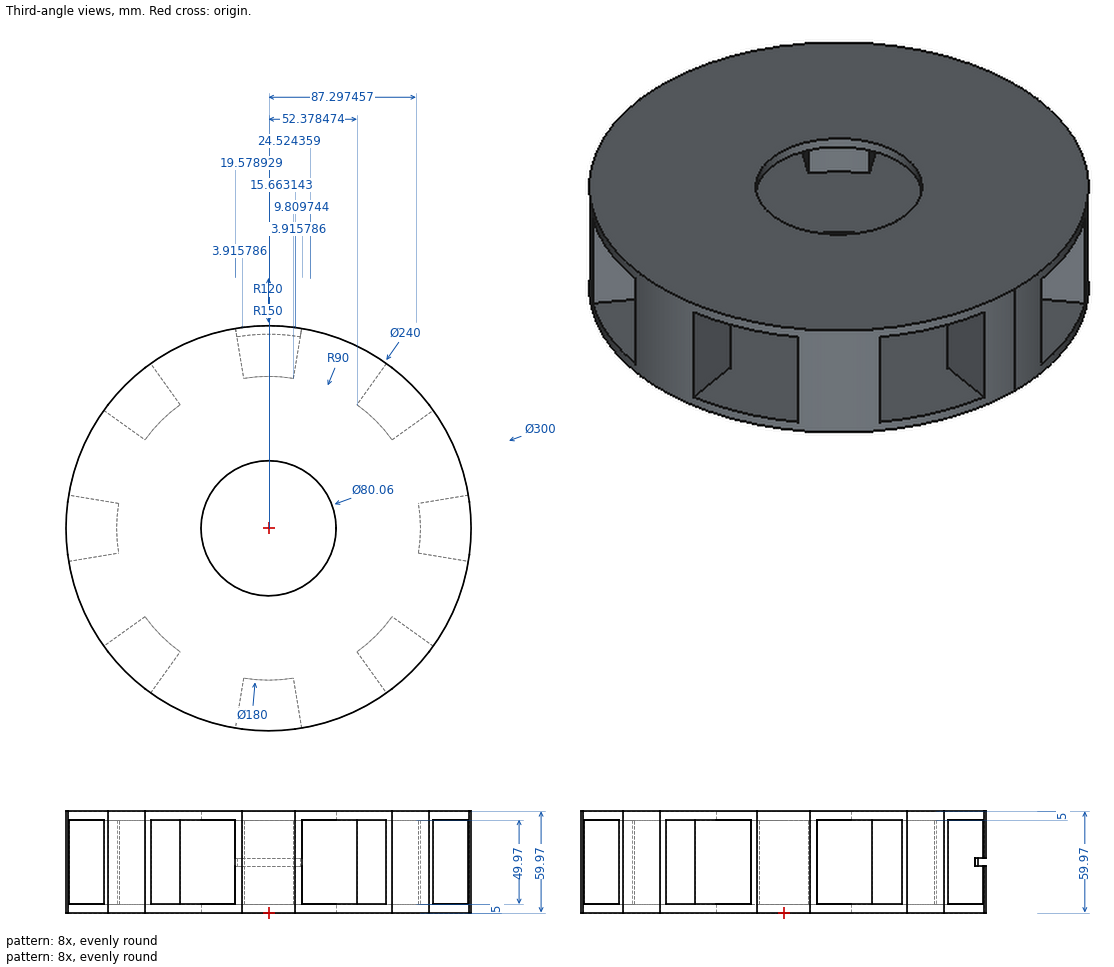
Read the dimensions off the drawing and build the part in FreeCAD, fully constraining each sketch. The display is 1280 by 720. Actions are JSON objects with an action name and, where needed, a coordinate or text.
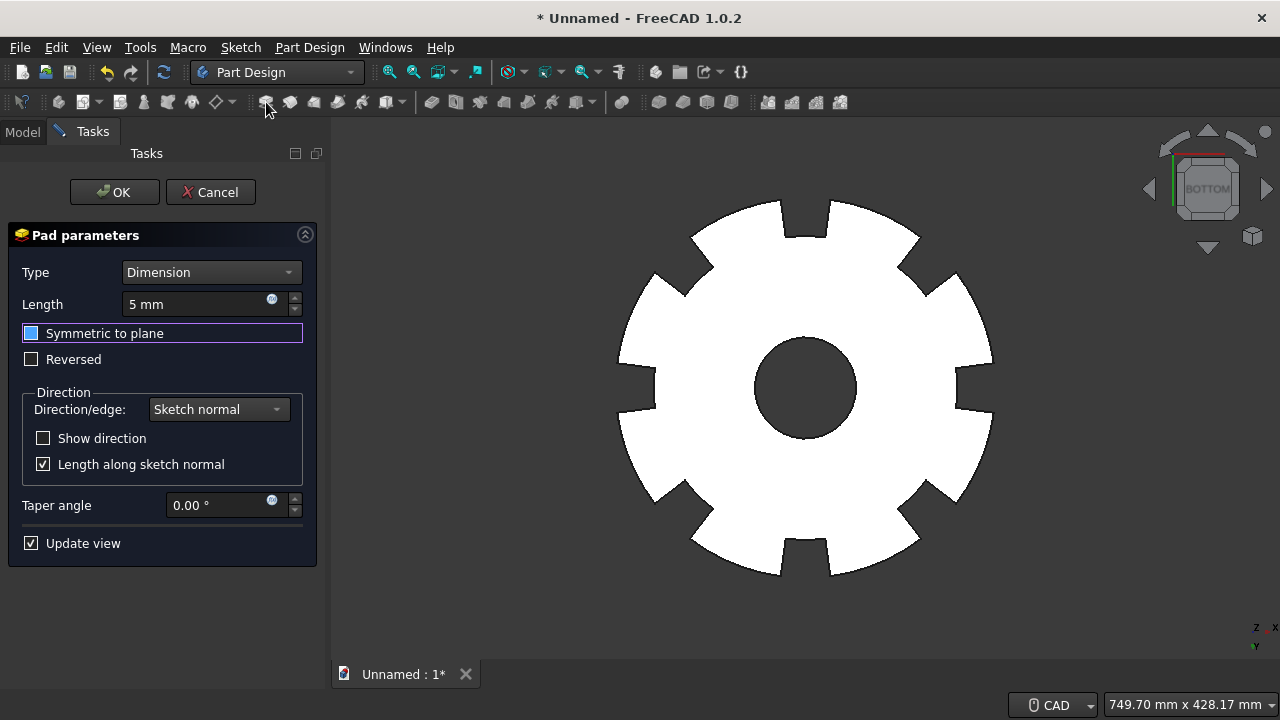
{"action": "left_click", "coordinate": [115, 192]}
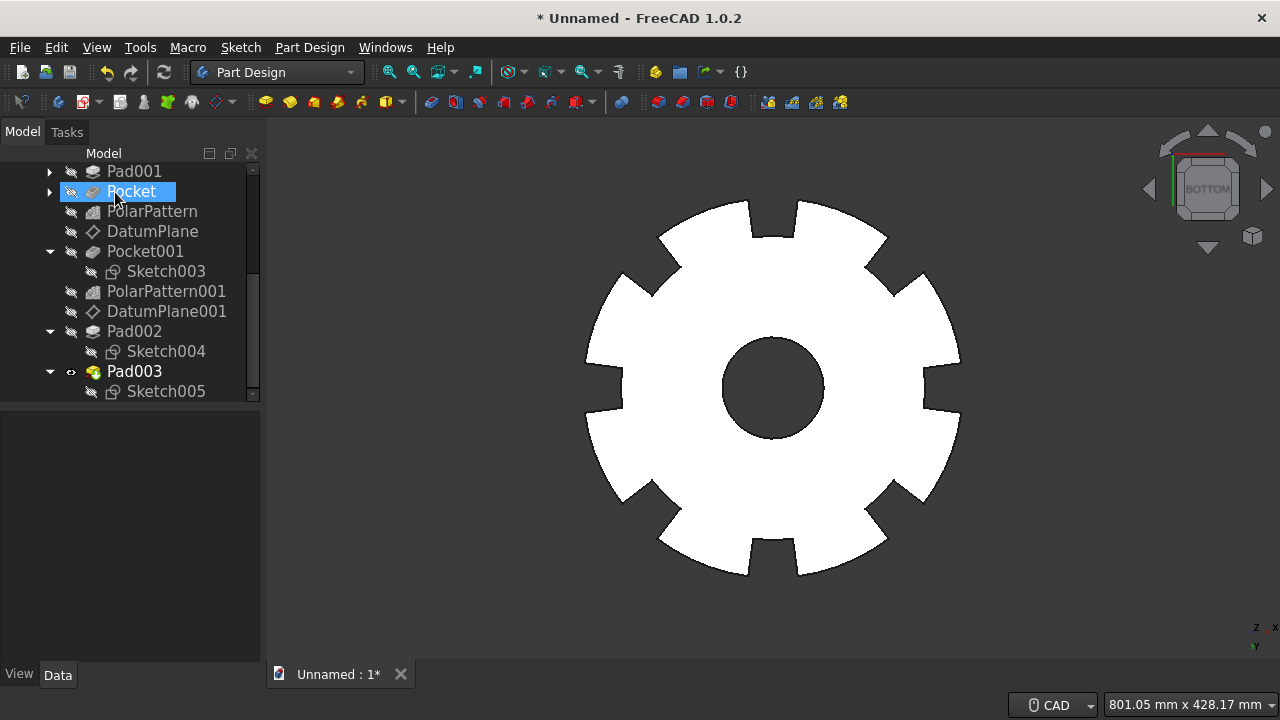
{"action": "left_click", "coordinate": [773, 495]}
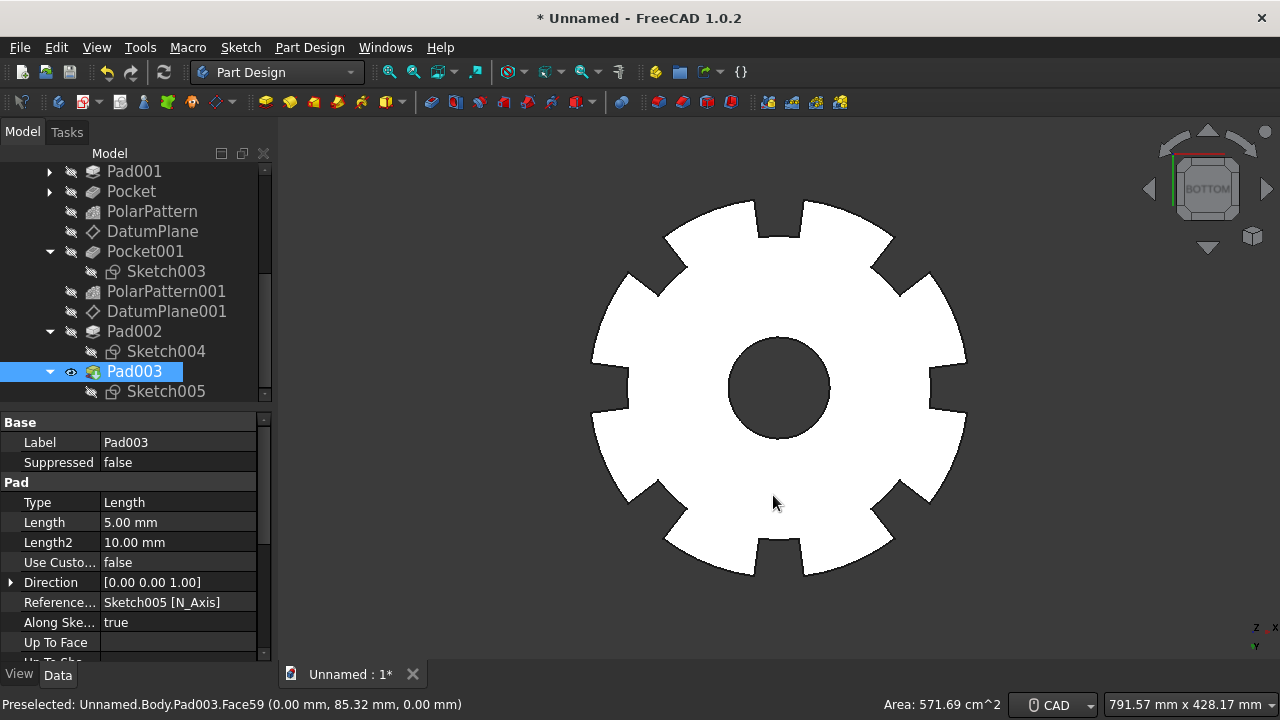
{"action": "left_click", "coordinate": [84, 102]}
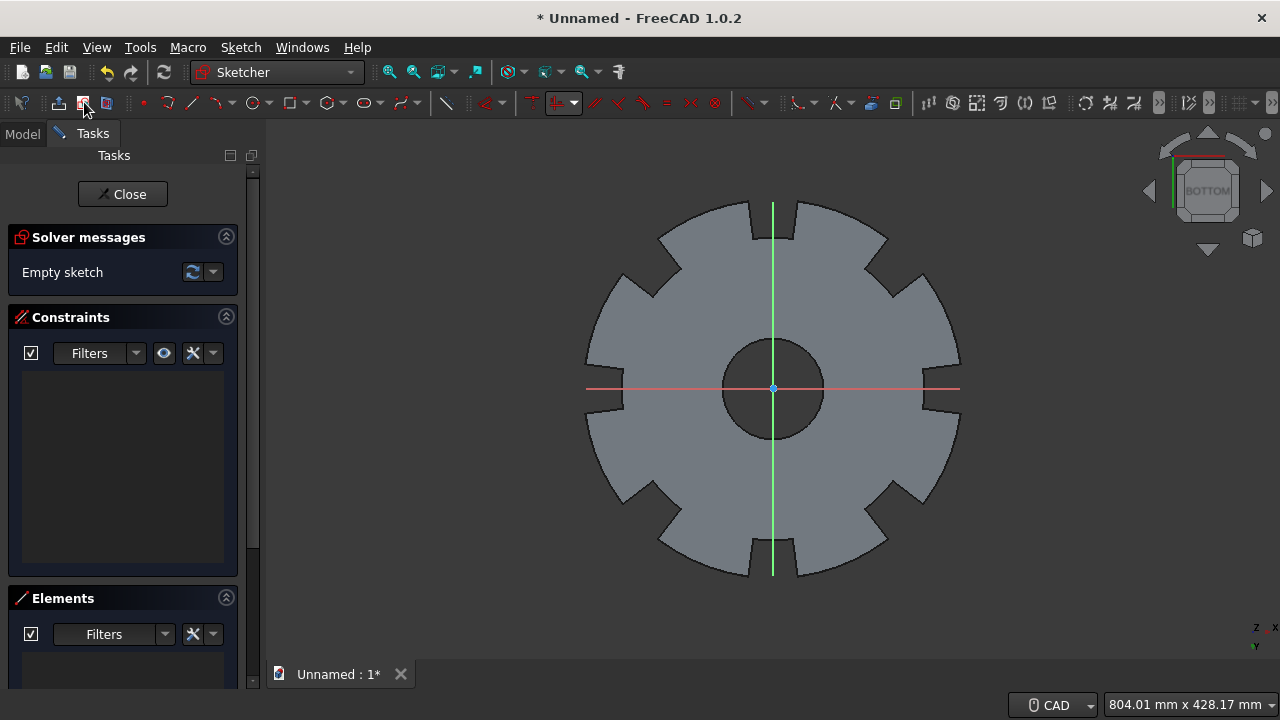
{"action": "key", "text": "g c"}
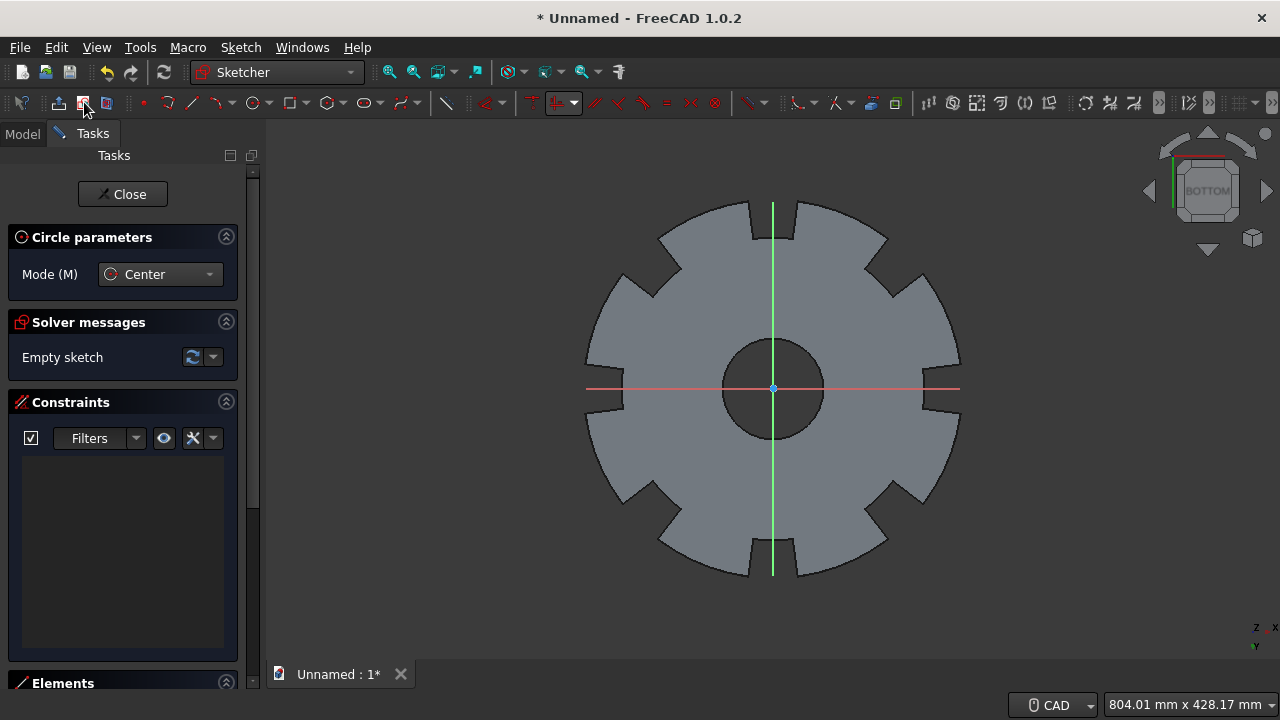
{"action": "left_click", "coordinate": [773, 389]}
{"action": "left_click", "coordinate": [907, 255]}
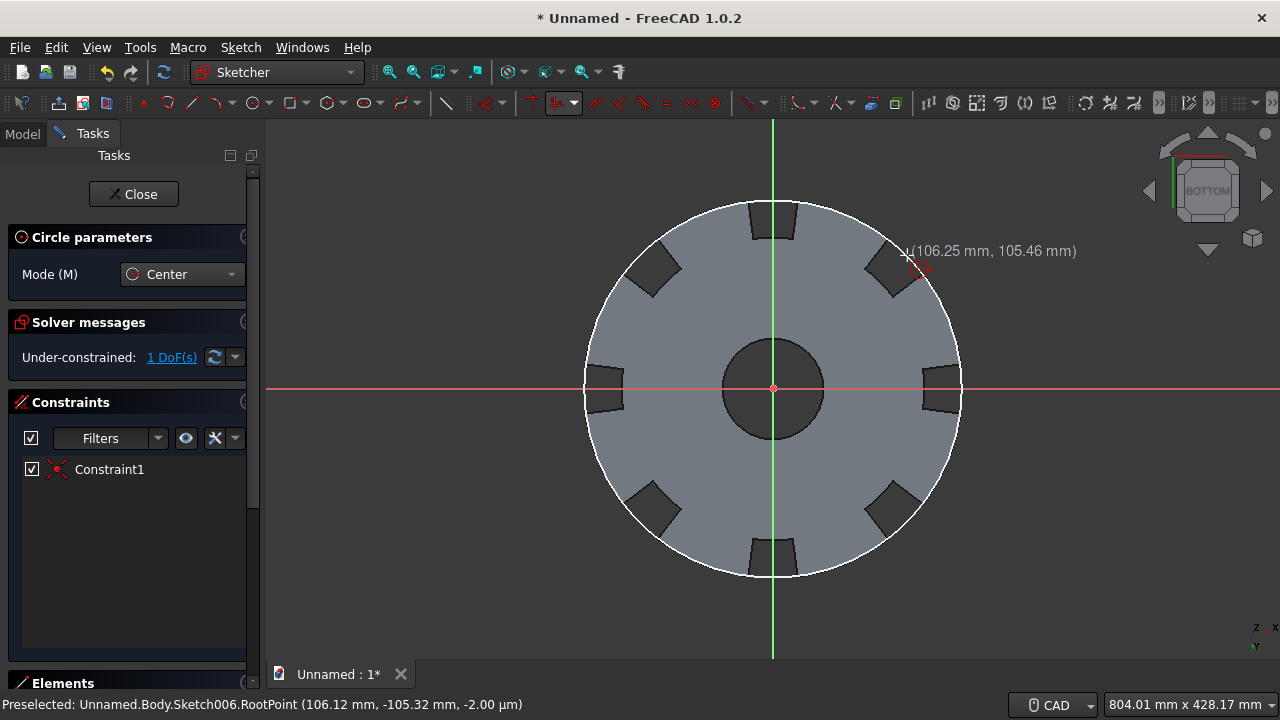
{"action": "left_click", "coordinate": [773, 389]}
{"action": "left_click", "coordinate": [880, 282]}
{"action": "key", "text": "Escape"}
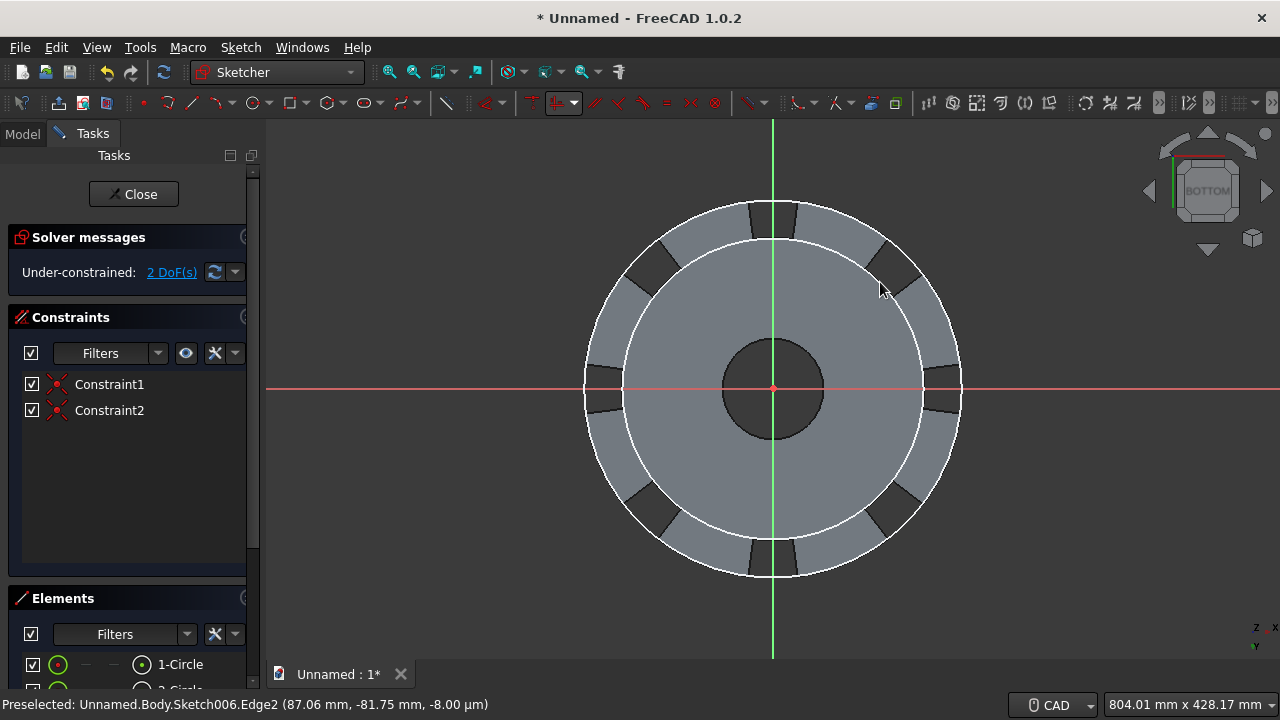
{"action": "left_click", "coordinate": [486, 104]}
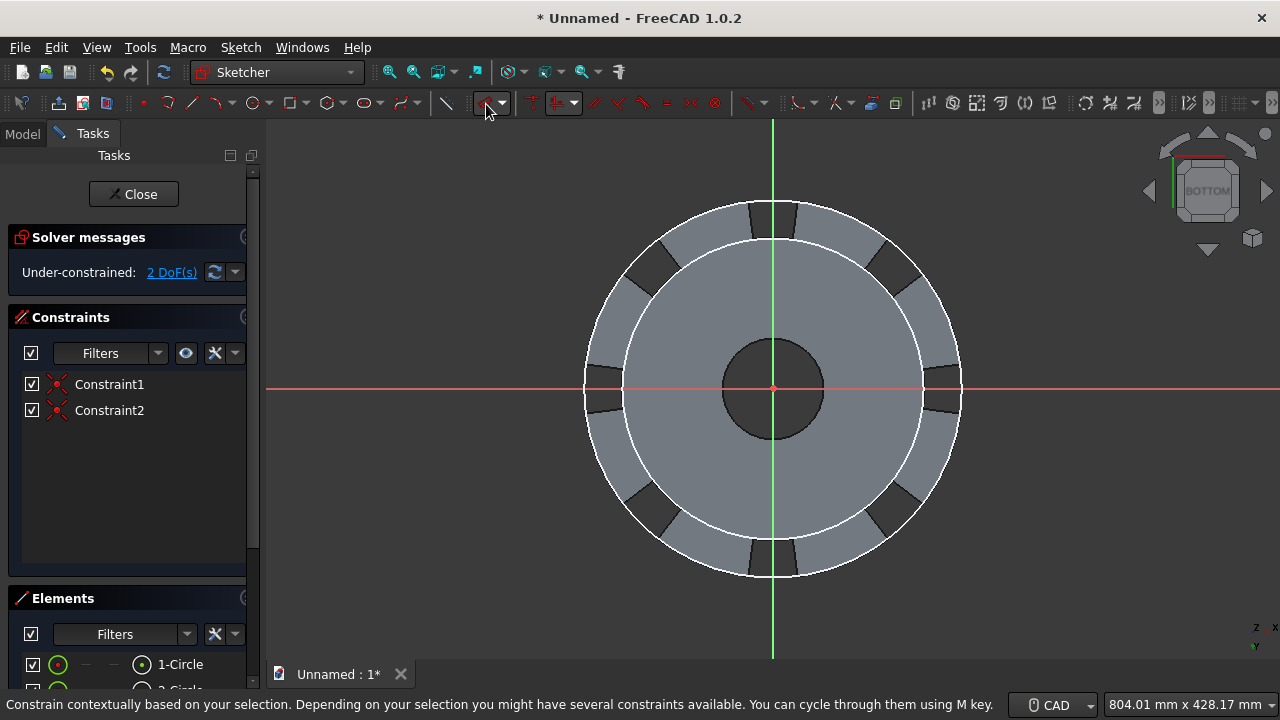
{"action": "left_click", "coordinate": [906, 255]}
{"action": "left_click", "coordinate": [929, 232]}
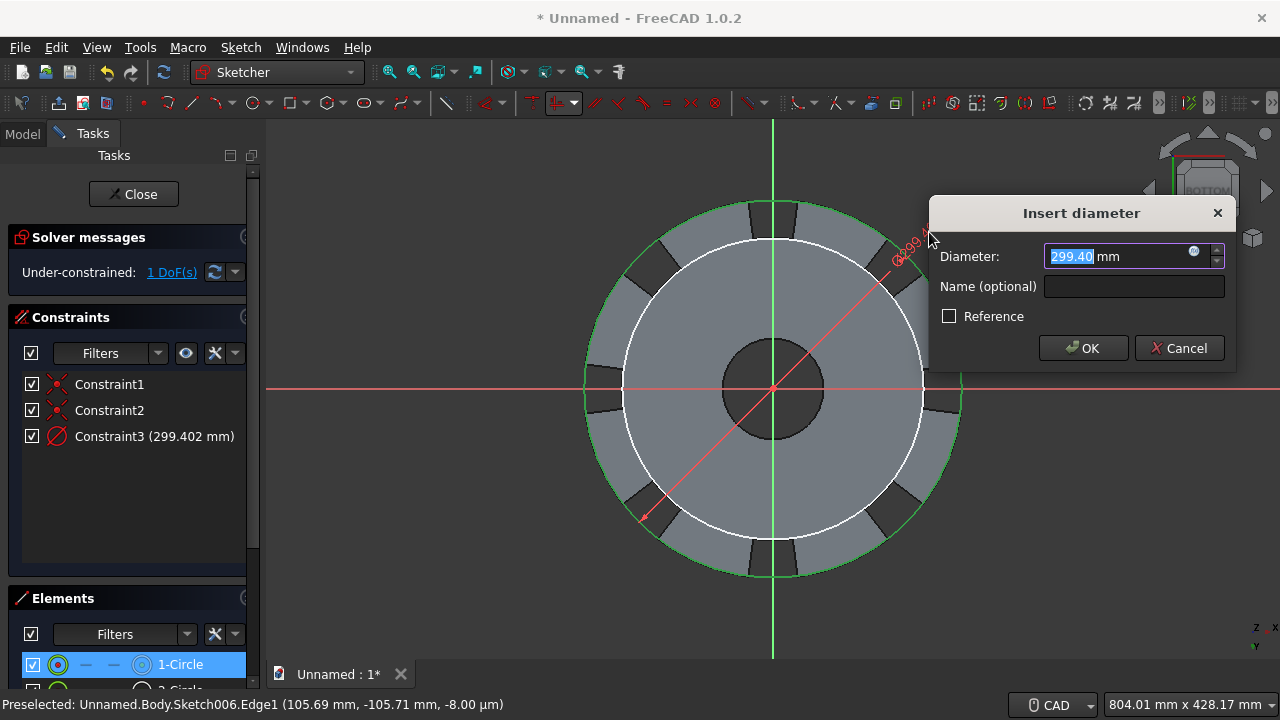
{"action": "type", "text": "300"}
{"action": "key", "text": "Return"}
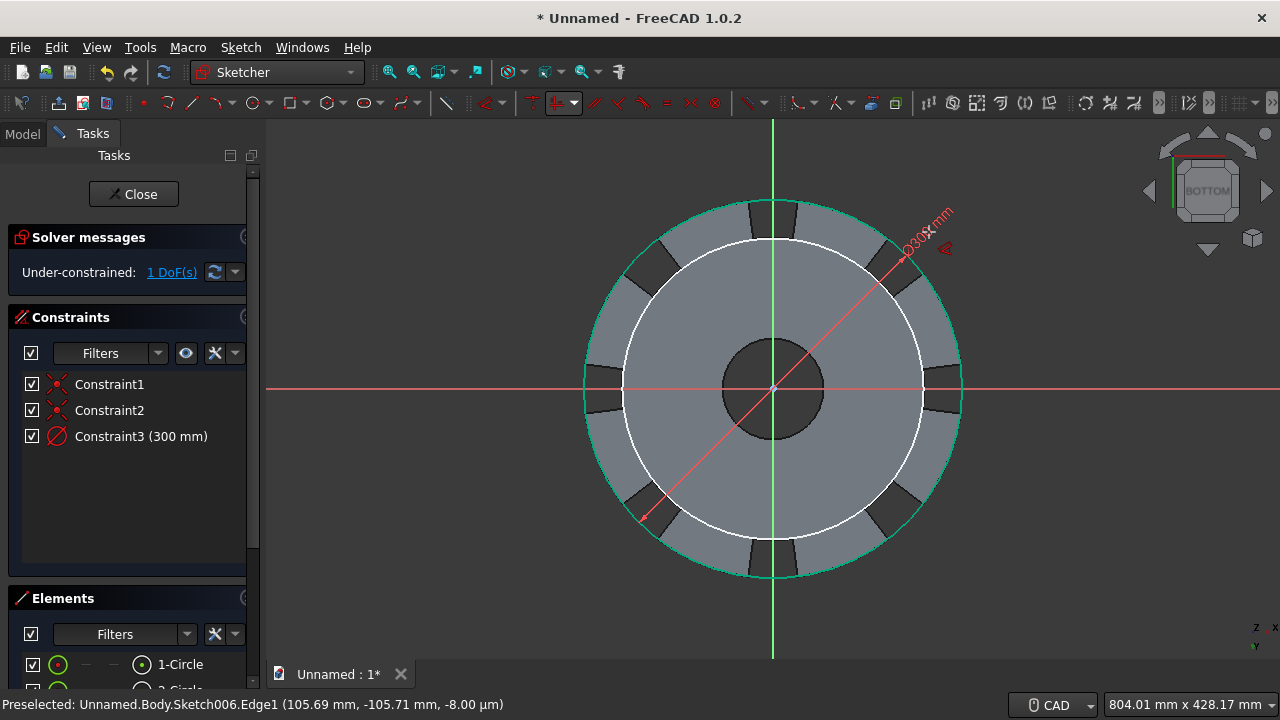
{"action": "left_click", "coordinate": [879, 282]}
{"action": "left_click", "coordinate": [970, 330]}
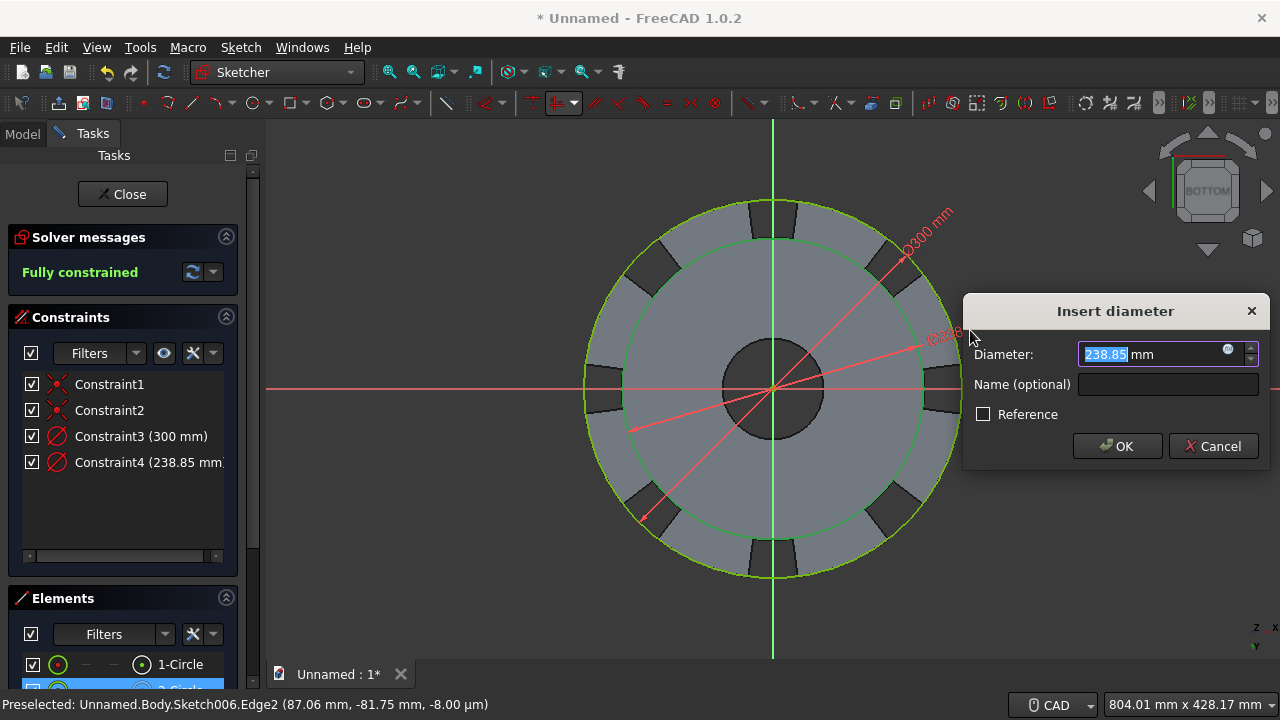
{"action": "type", "text": "240"}
{"action": "key", "text": "Return"}
{"action": "key", "text": "Escape"}